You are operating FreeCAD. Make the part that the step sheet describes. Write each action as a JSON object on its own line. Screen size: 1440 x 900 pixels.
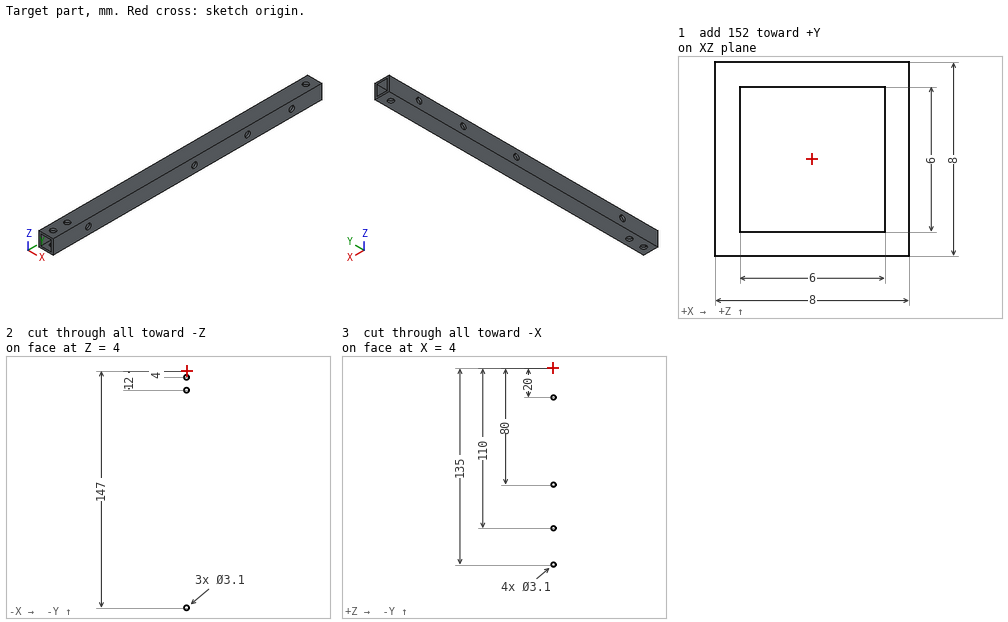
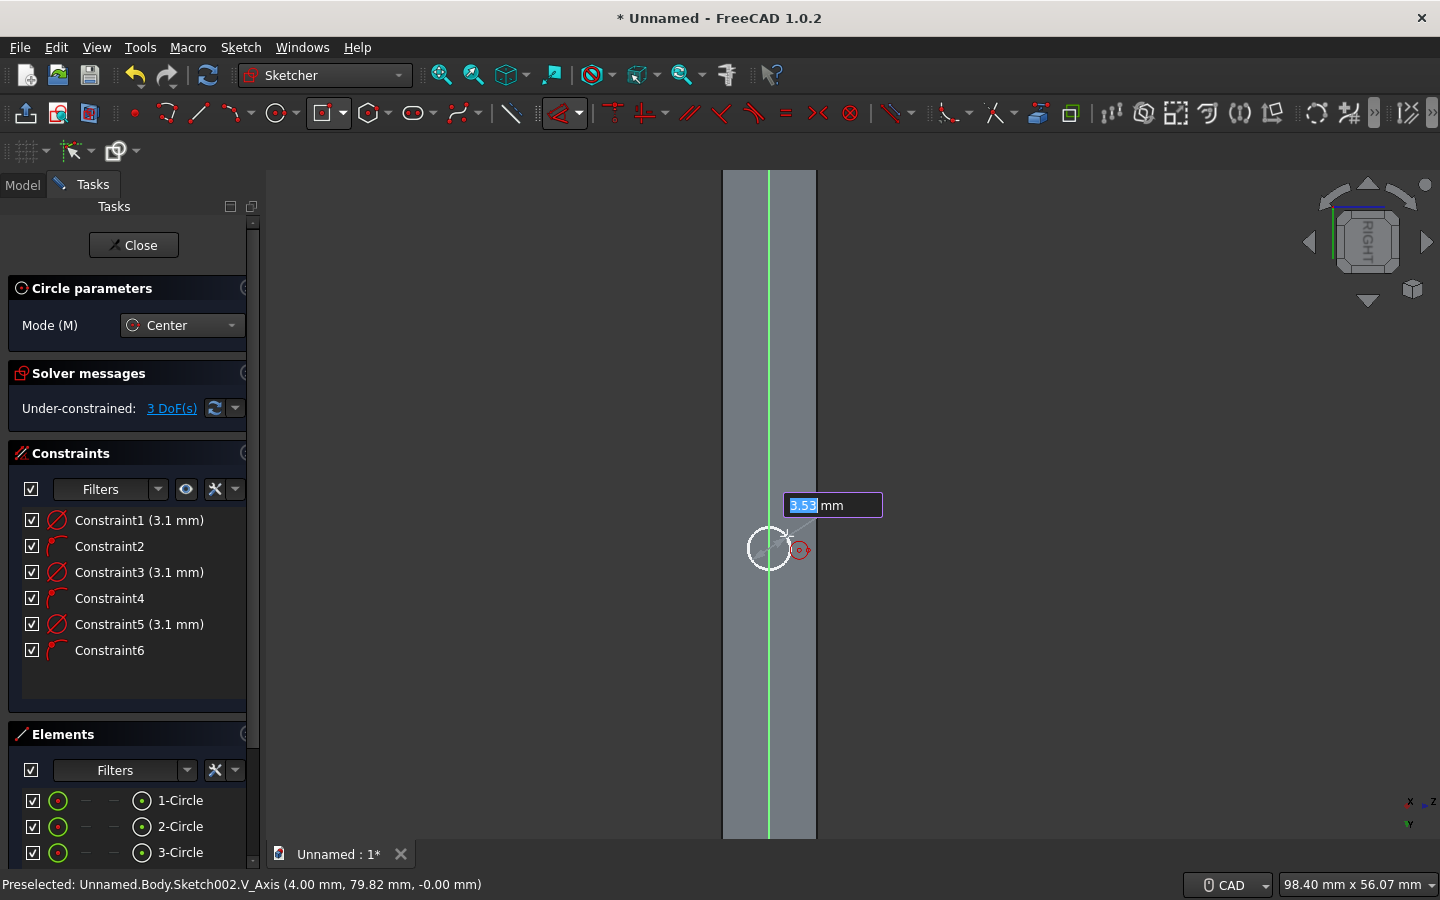
{"action": "type", "text": "3.1"}
{"action": "key", "text": "Return"}
{"action": "key", "text": "Escape"}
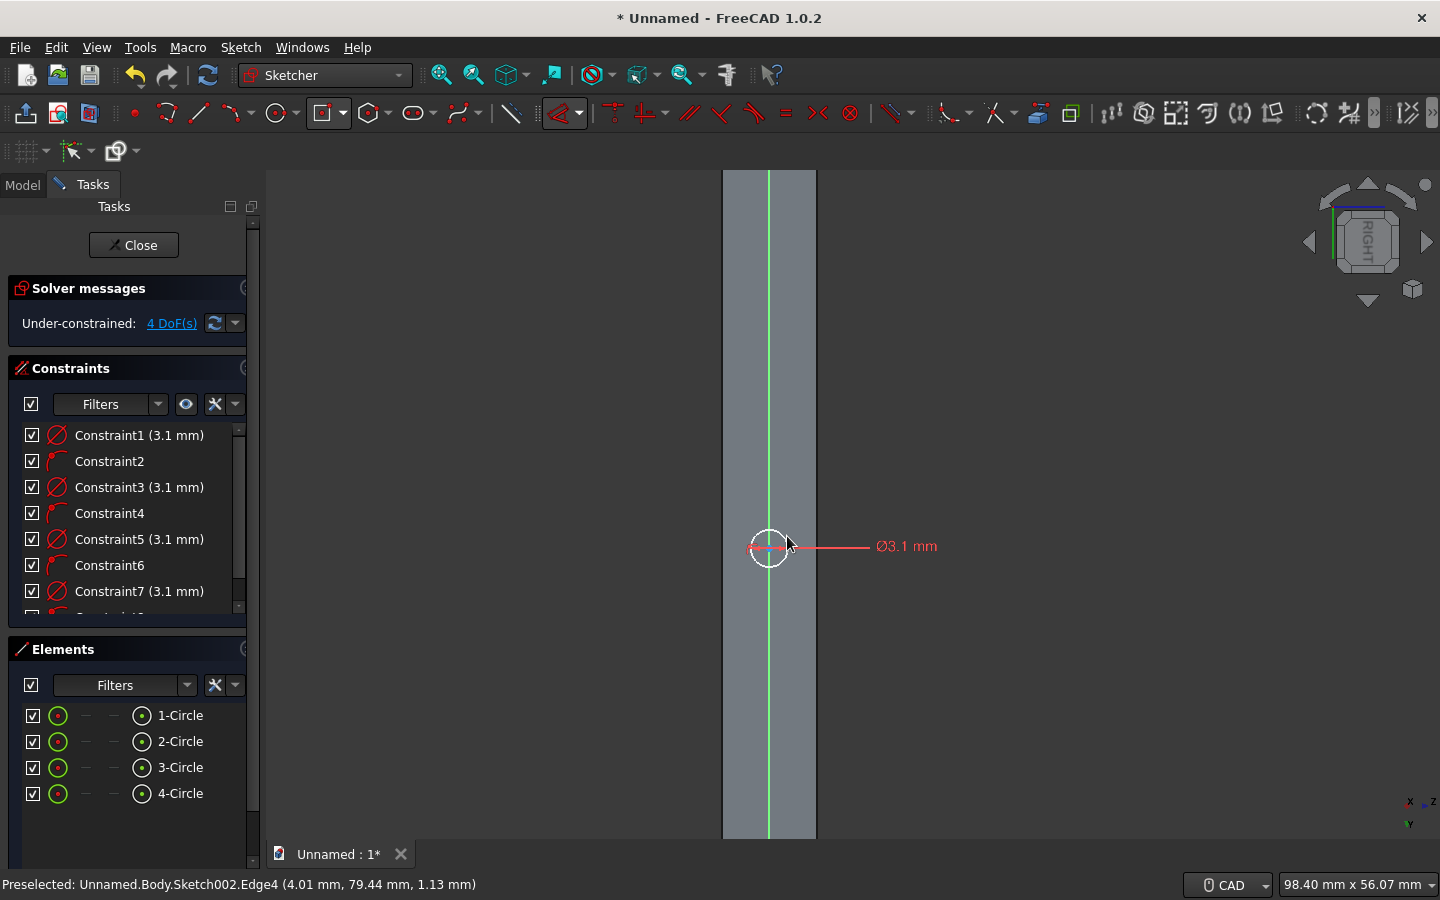
{"action": "scroll", "coordinate": [789, 538], "scroll_direction": "down", "scroll_amount": 7}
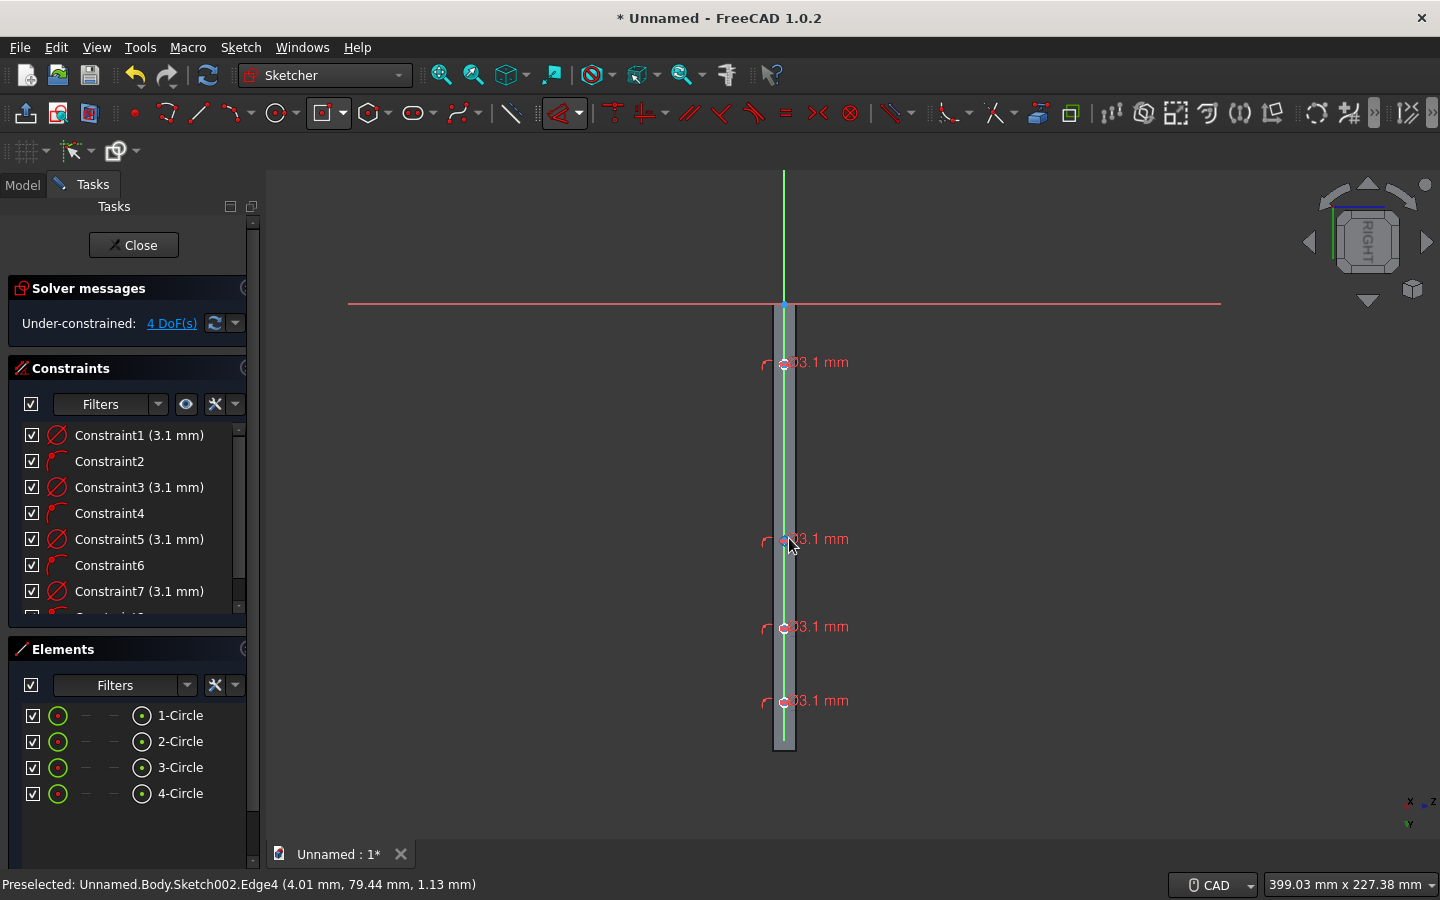
{"action": "left_click", "coordinate": [784, 364]}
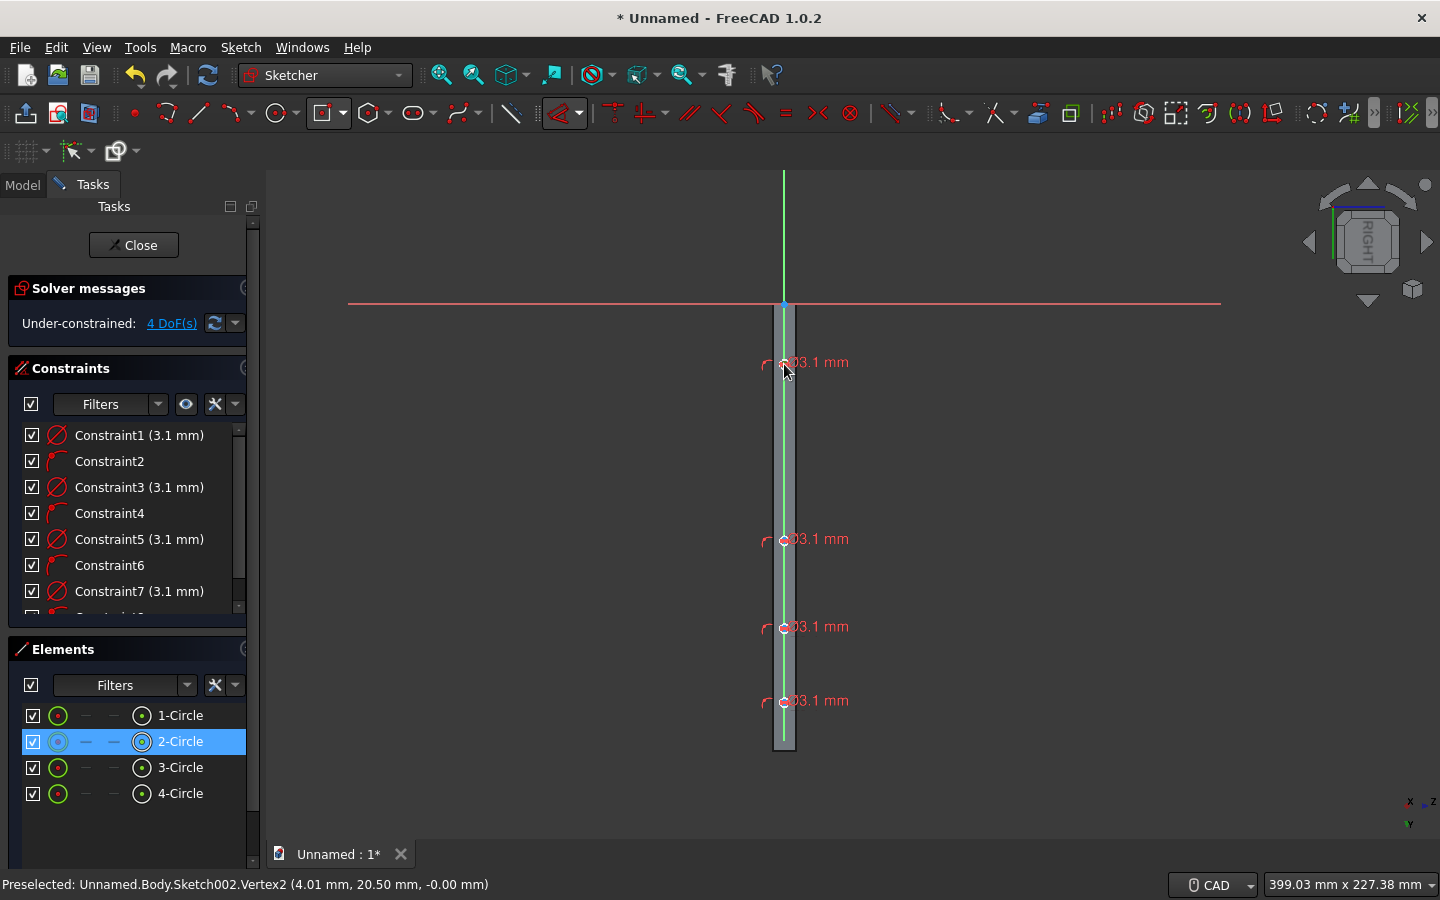
{"action": "left_click", "coordinate": [582, 114]}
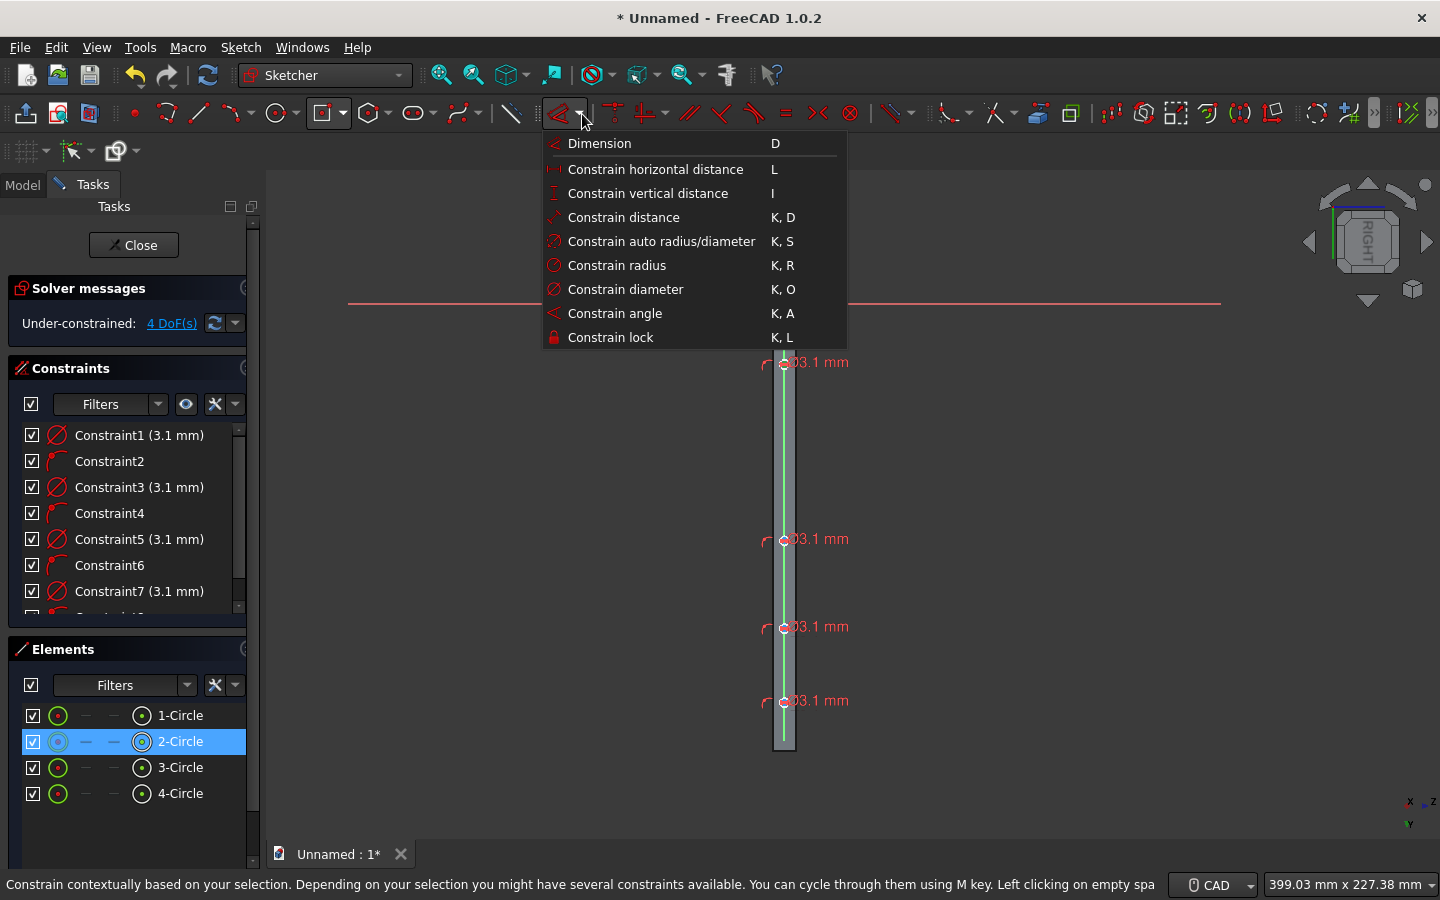
{"action": "left_click", "coordinate": [695, 193]}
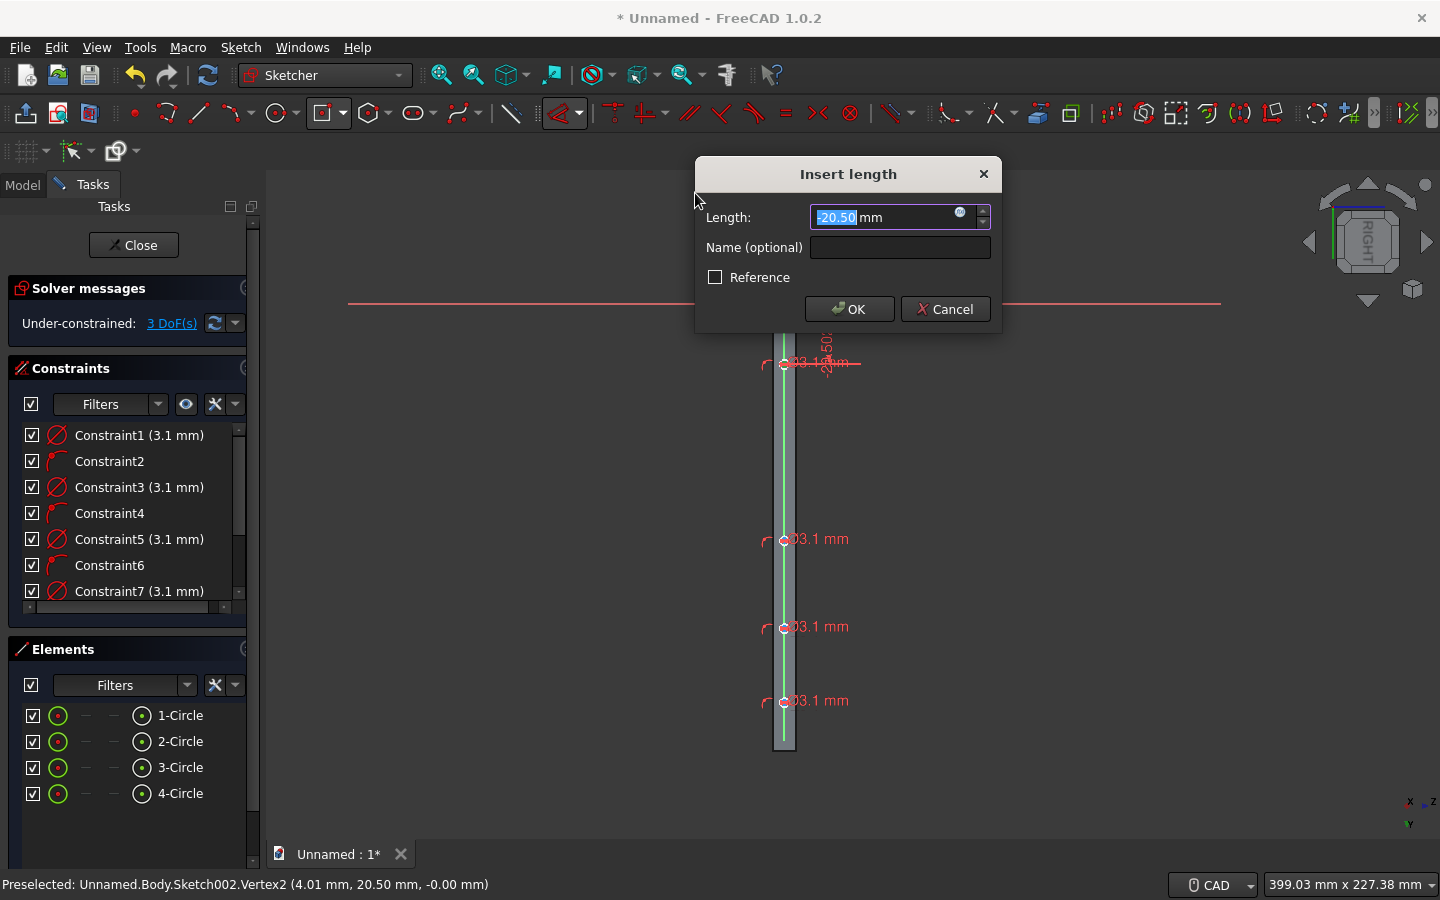
{"action": "type", "text": "-20"}
{"action": "key", "text": "Return"}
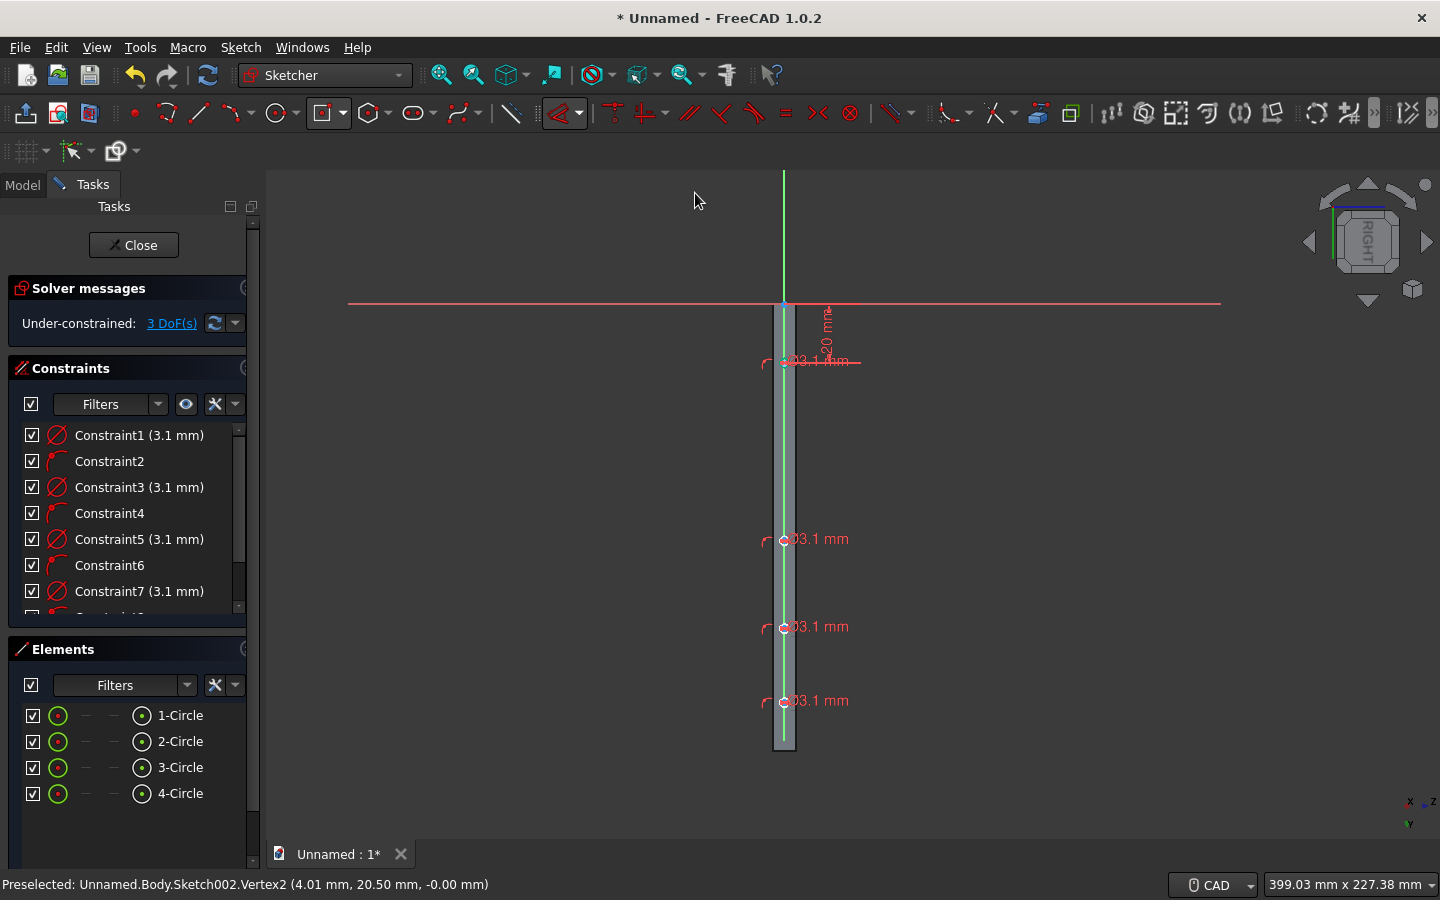
{"action": "left_click", "coordinate": [784, 541]}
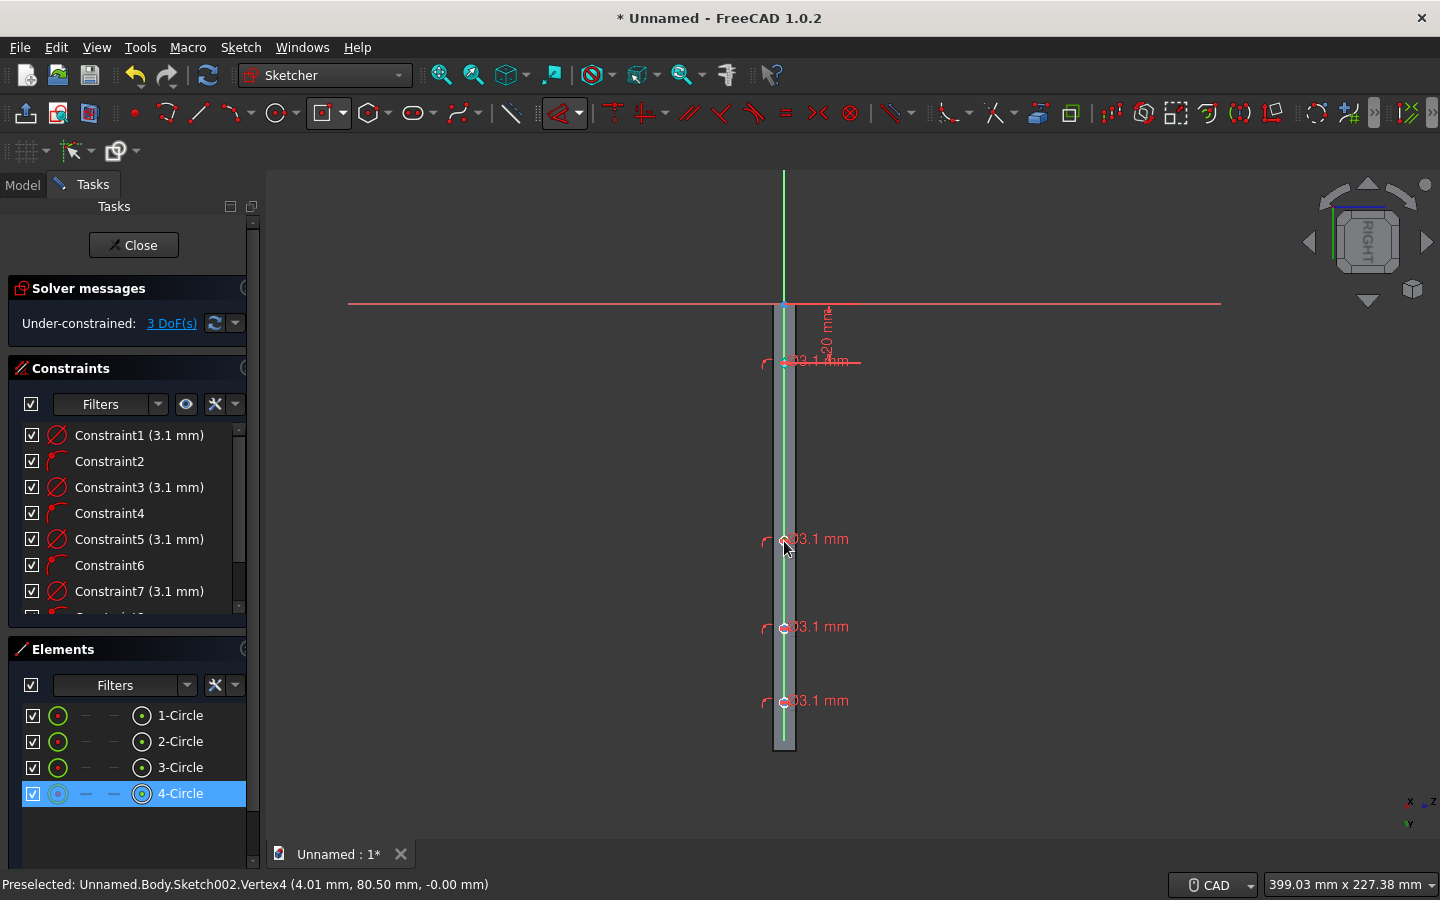
{"action": "left_click", "coordinate": [582, 114]}